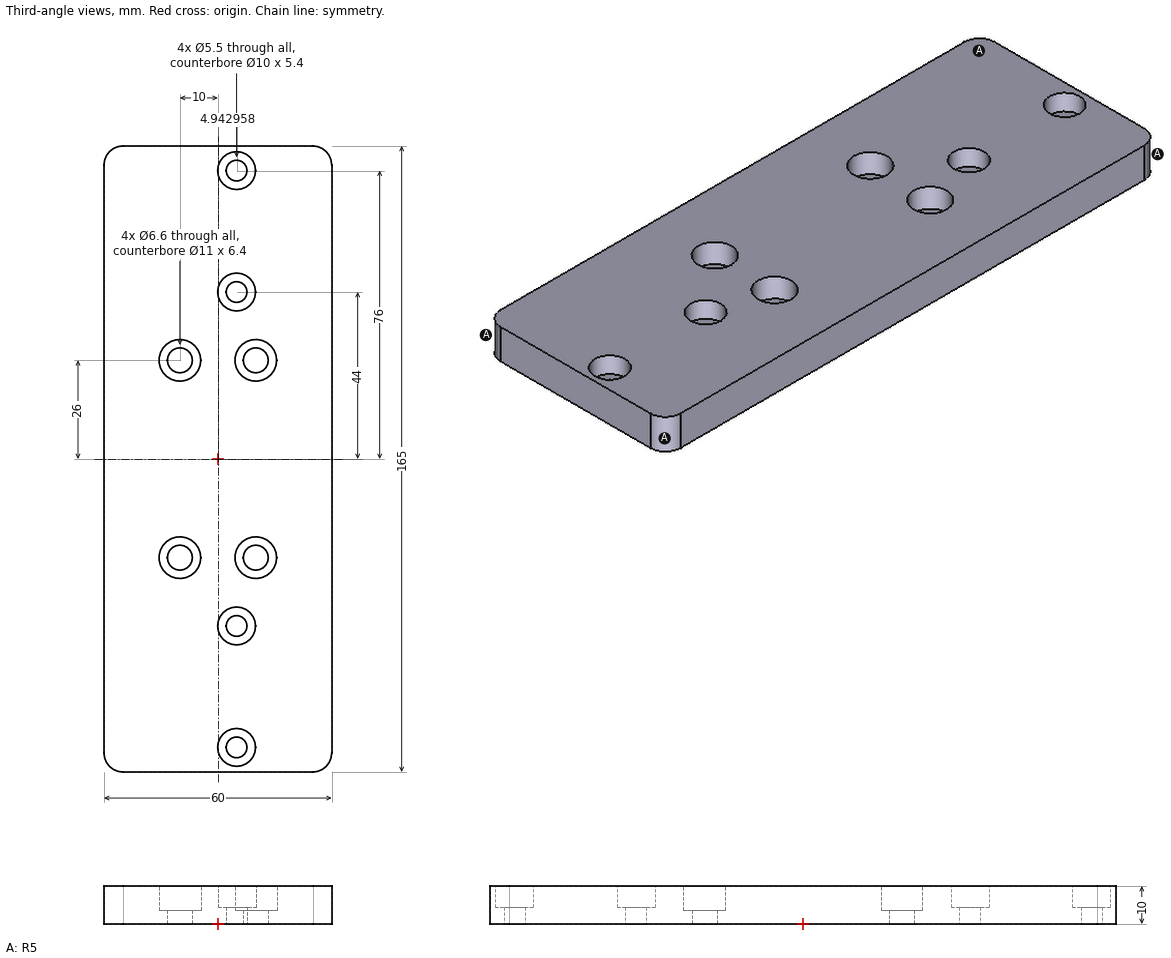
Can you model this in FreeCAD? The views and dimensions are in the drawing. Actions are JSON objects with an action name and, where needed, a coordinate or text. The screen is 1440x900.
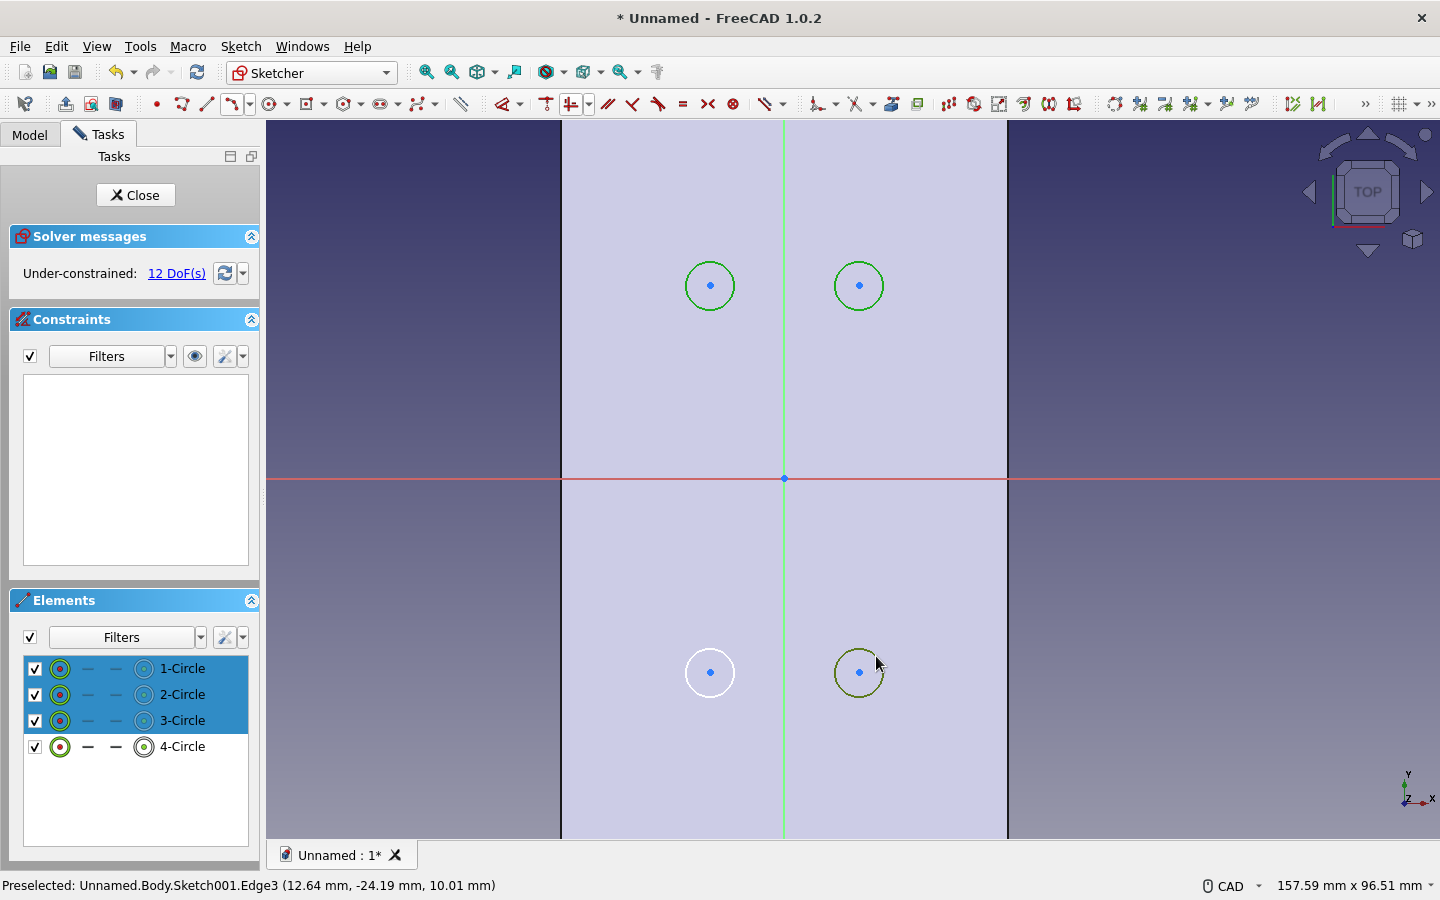
{"action": "left_click", "coordinate": [727, 656]}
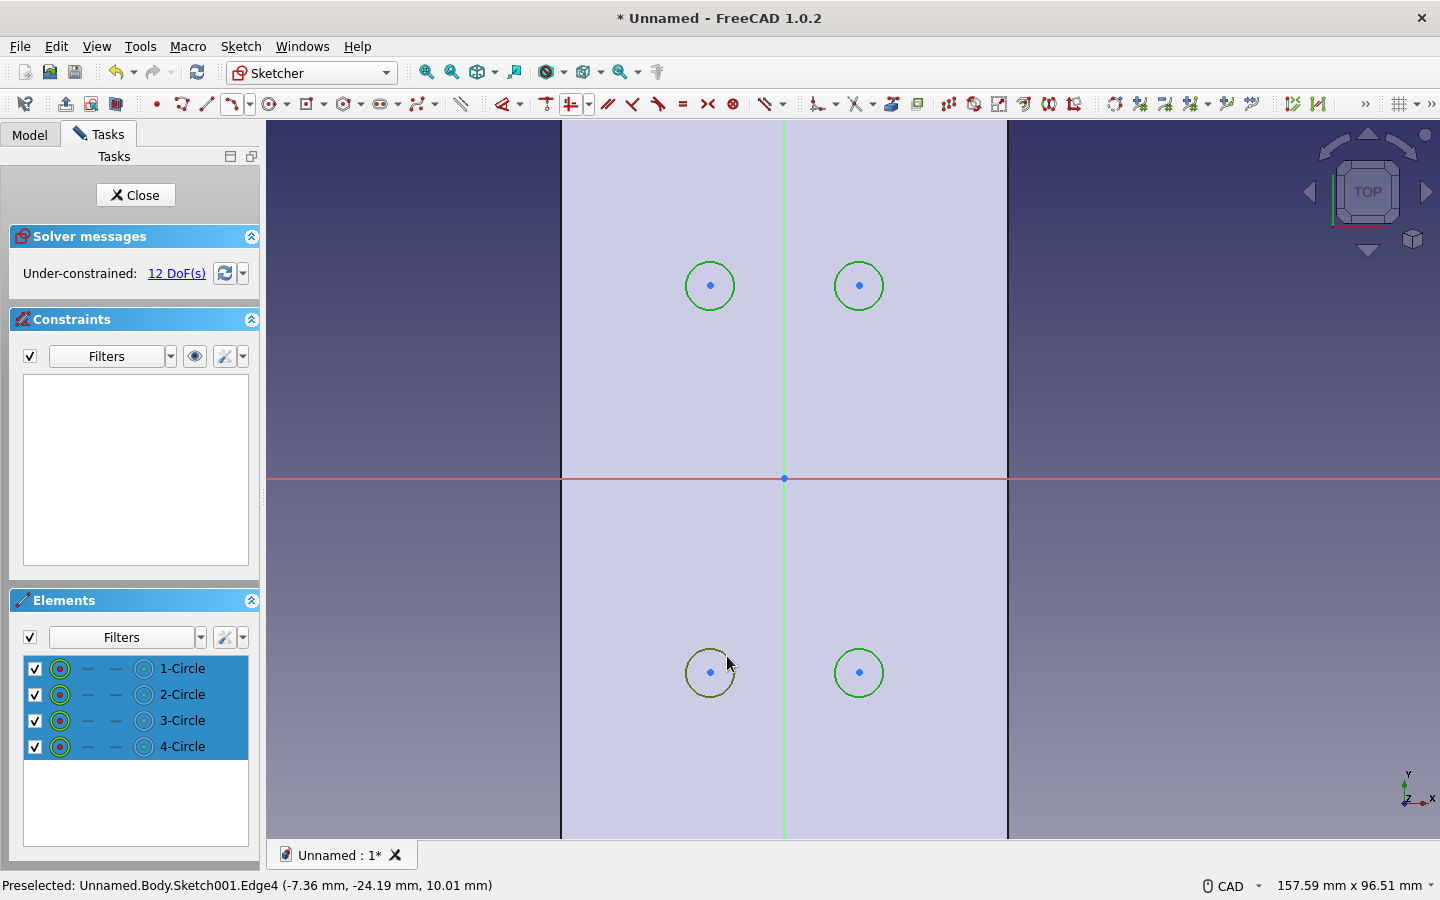
{"action": "left_click", "coordinate": [683, 104]}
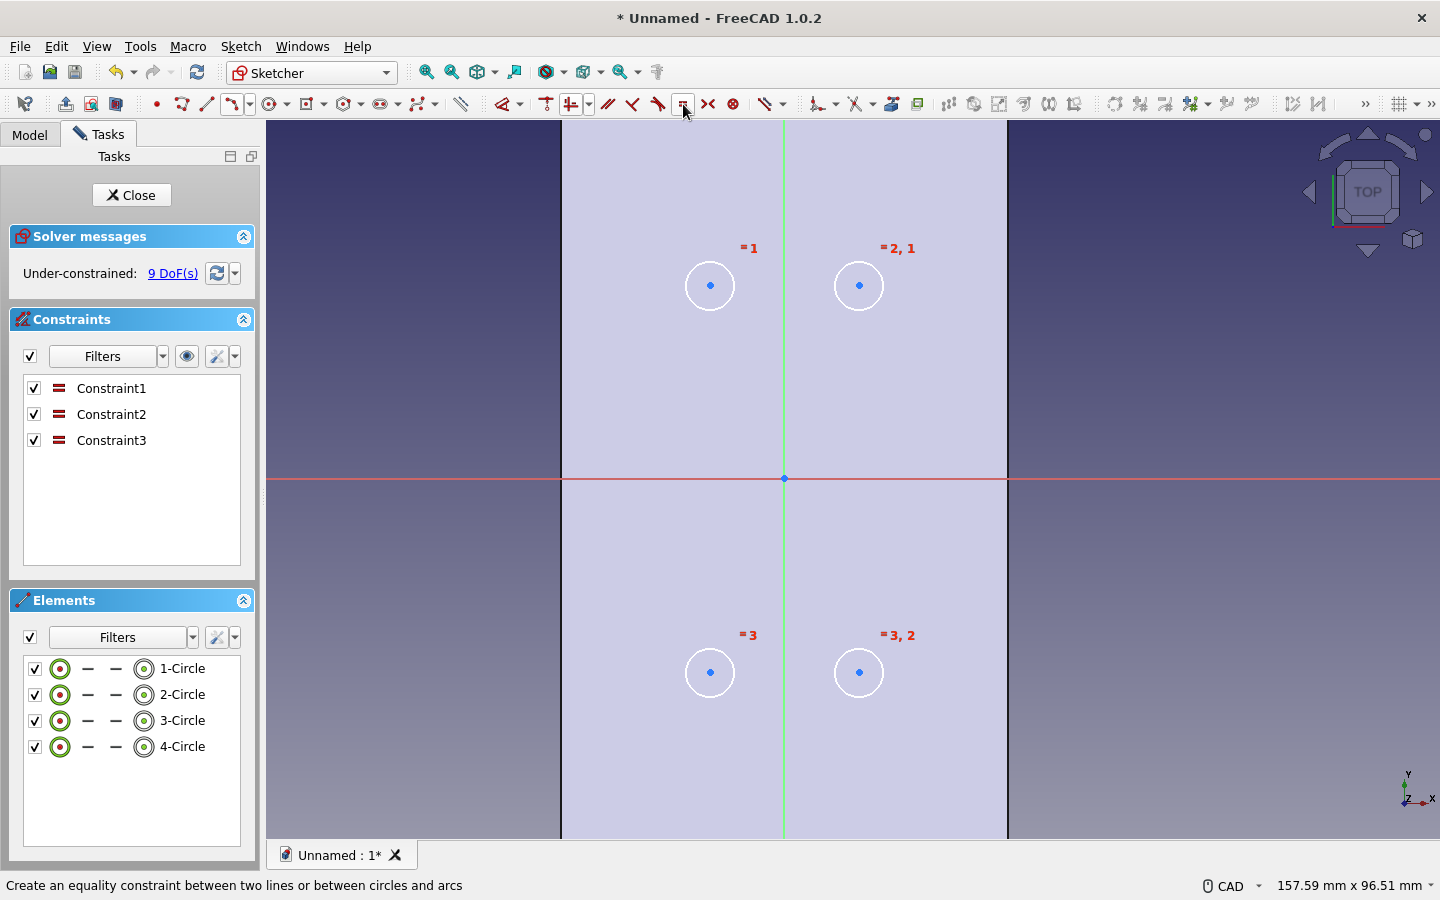
{"action": "left_click", "coordinate": [710, 286]}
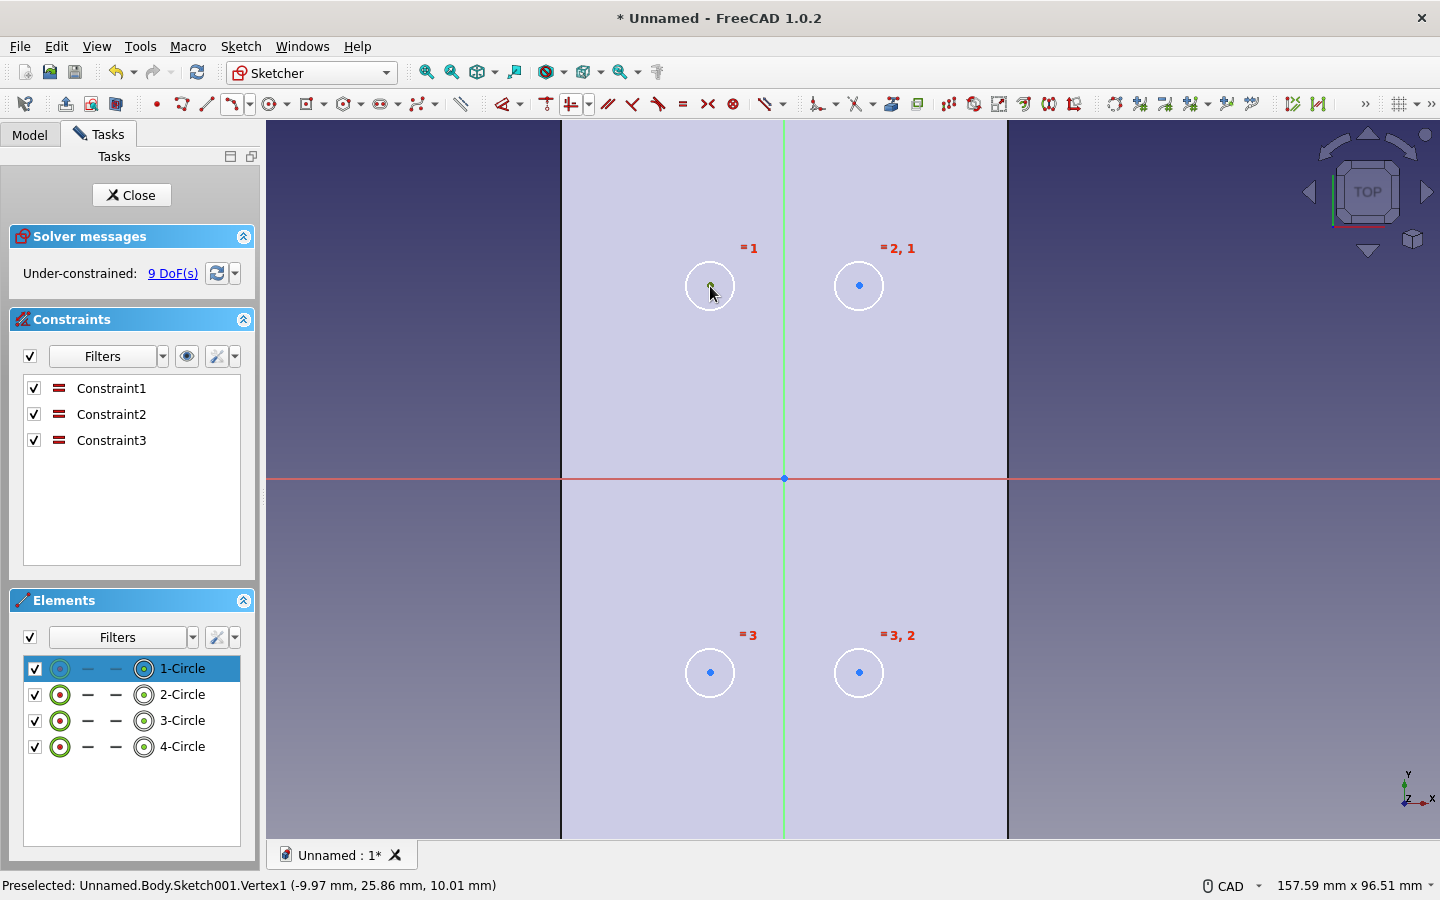
{"action": "left_click", "coordinate": [859, 286]}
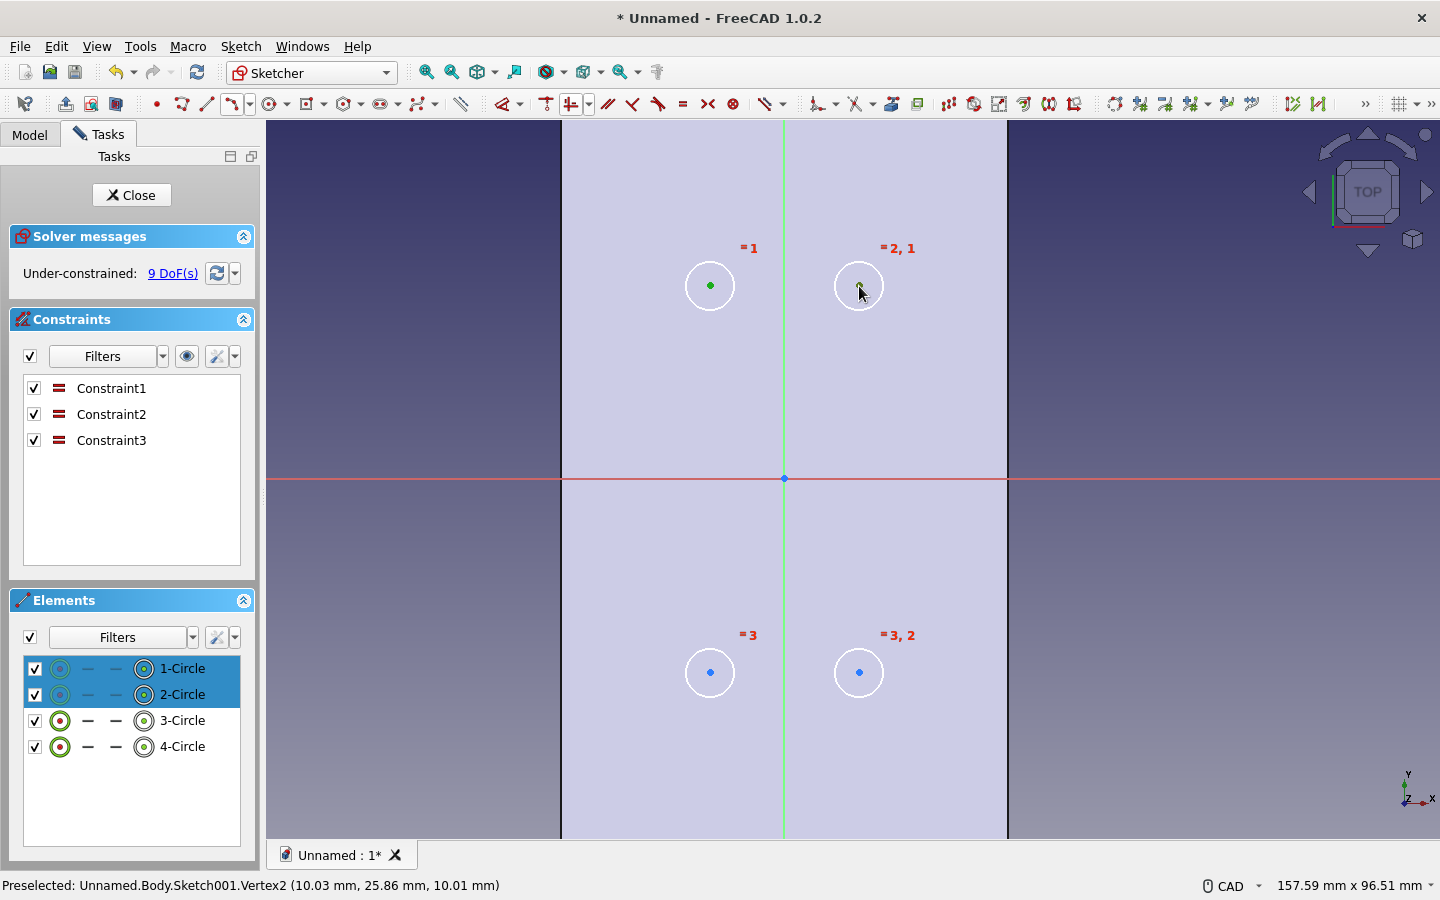
{"action": "left_click", "coordinate": [784, 764]}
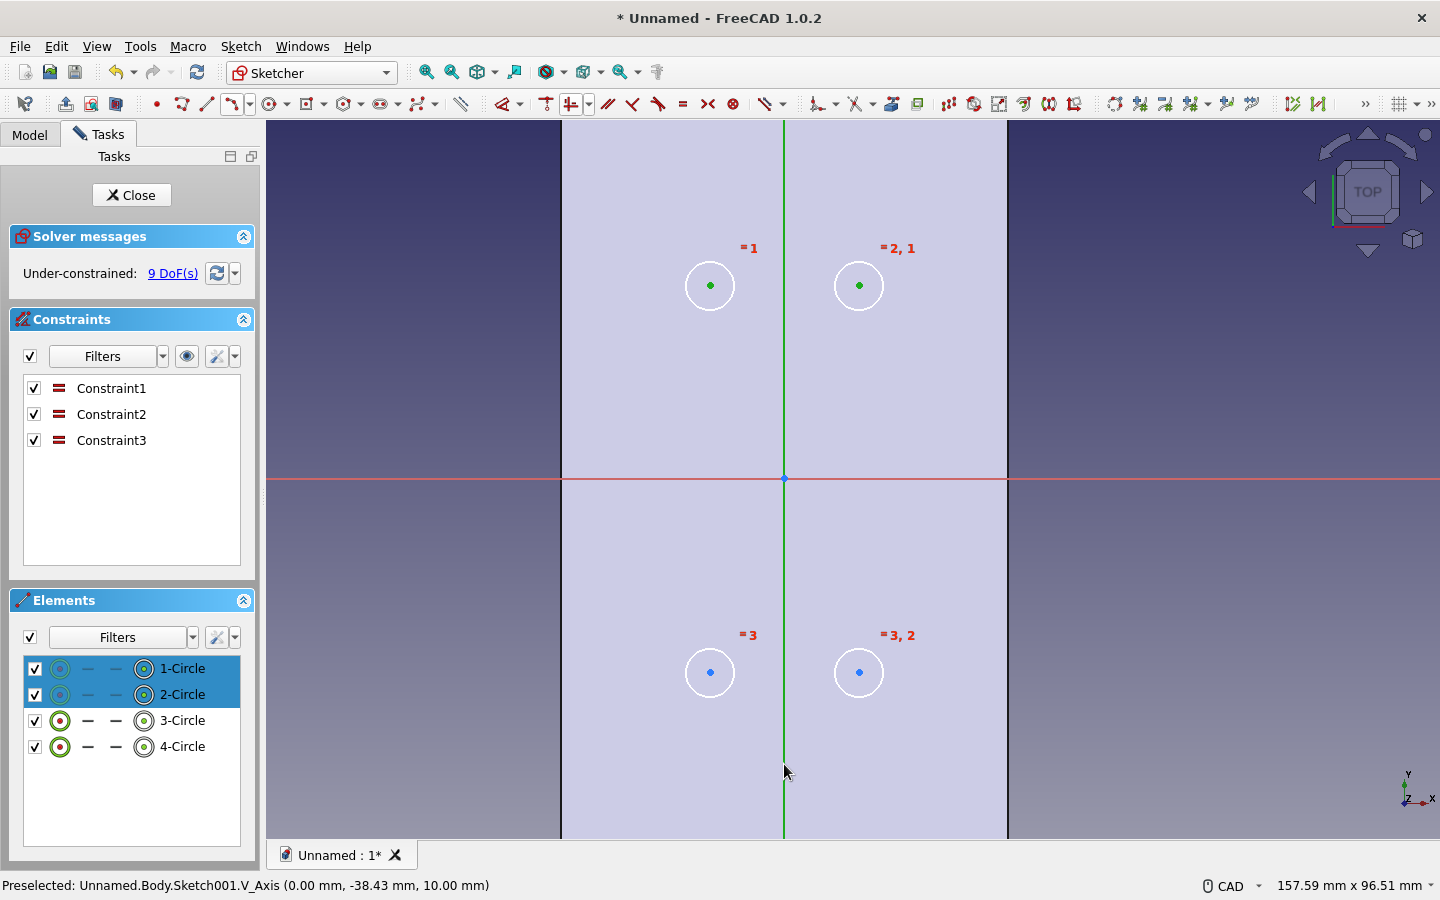
{"action": "left_click", "coordinate": [708, 104]}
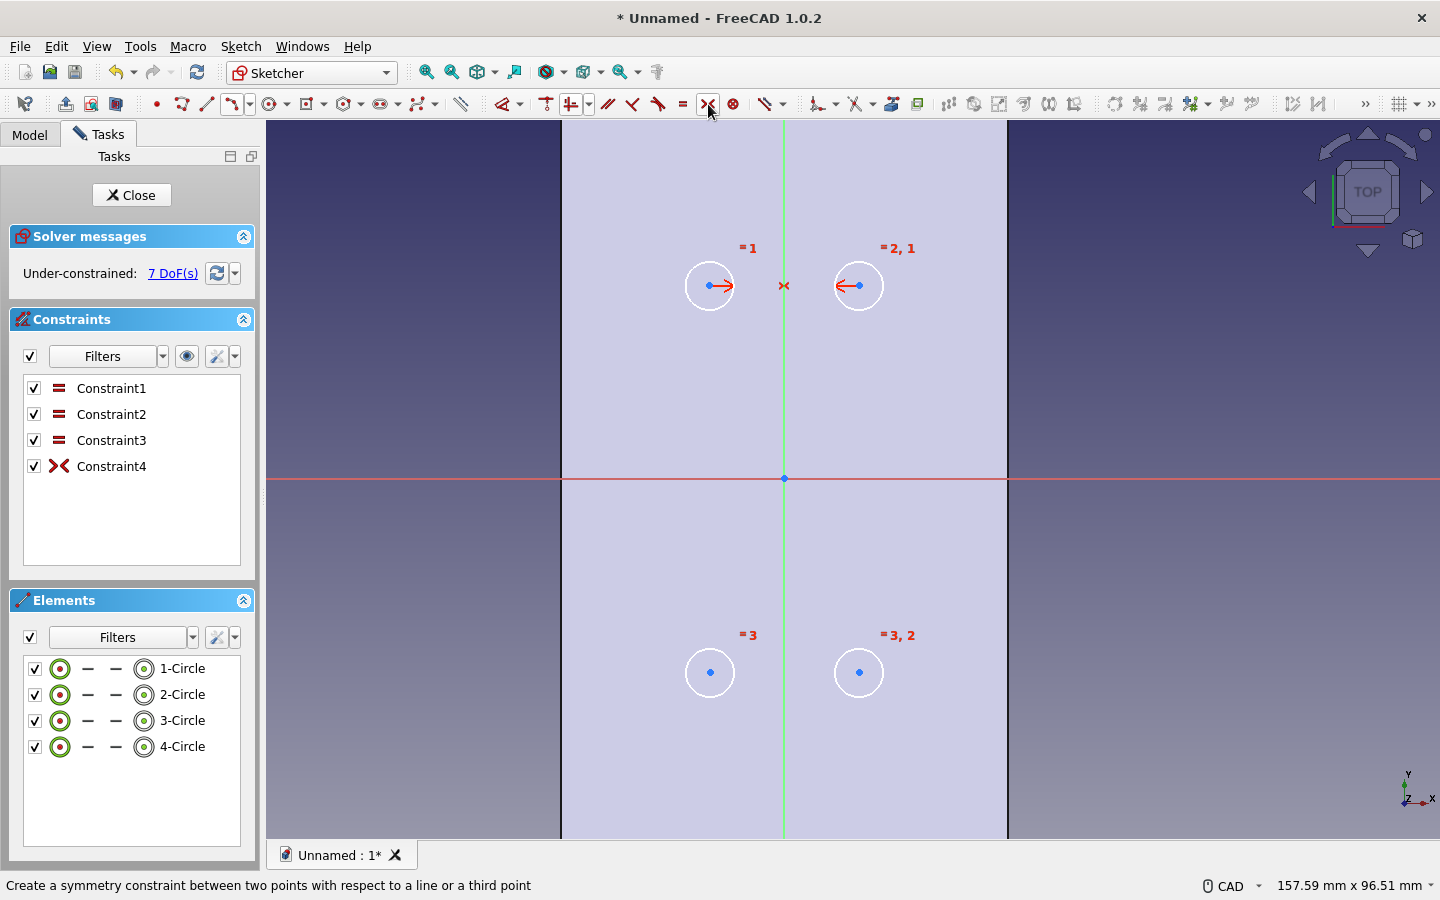
{"action": "left_click", "coordinate": [859, 286]}